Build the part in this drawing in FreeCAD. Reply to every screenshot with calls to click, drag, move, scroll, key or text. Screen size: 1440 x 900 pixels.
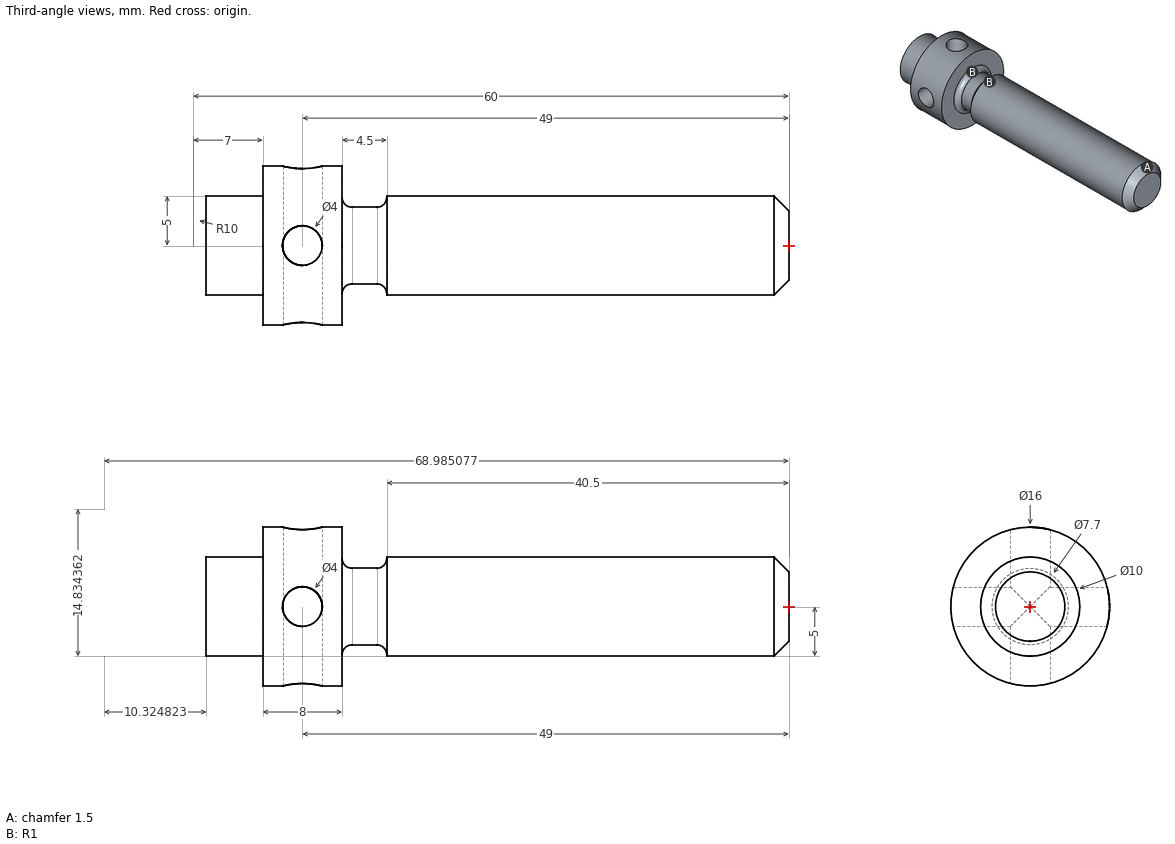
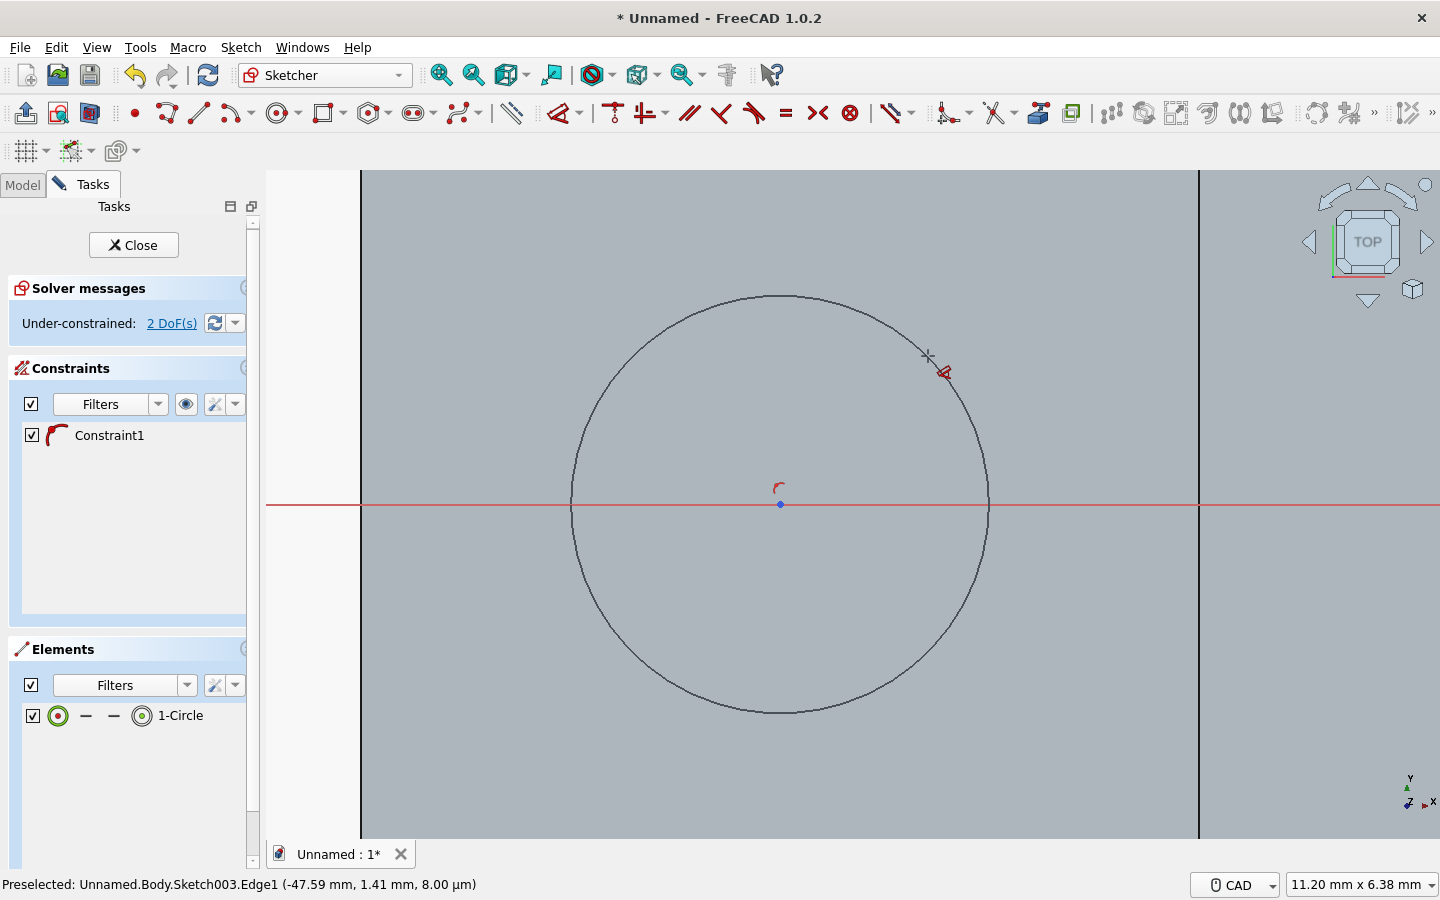
click(927, 356)
click(950, 333)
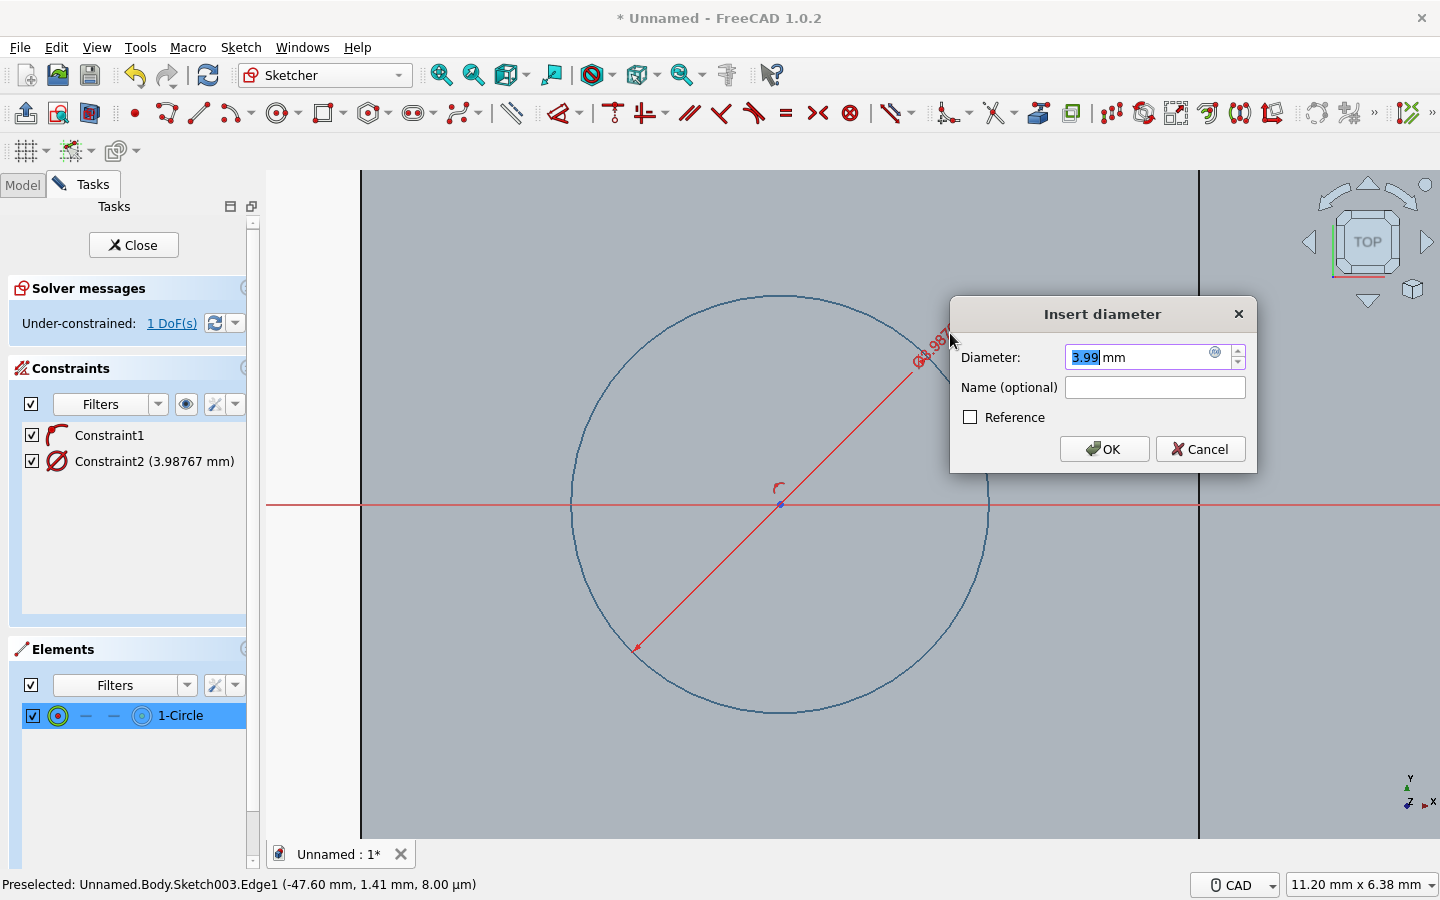
text(4)
key(Return)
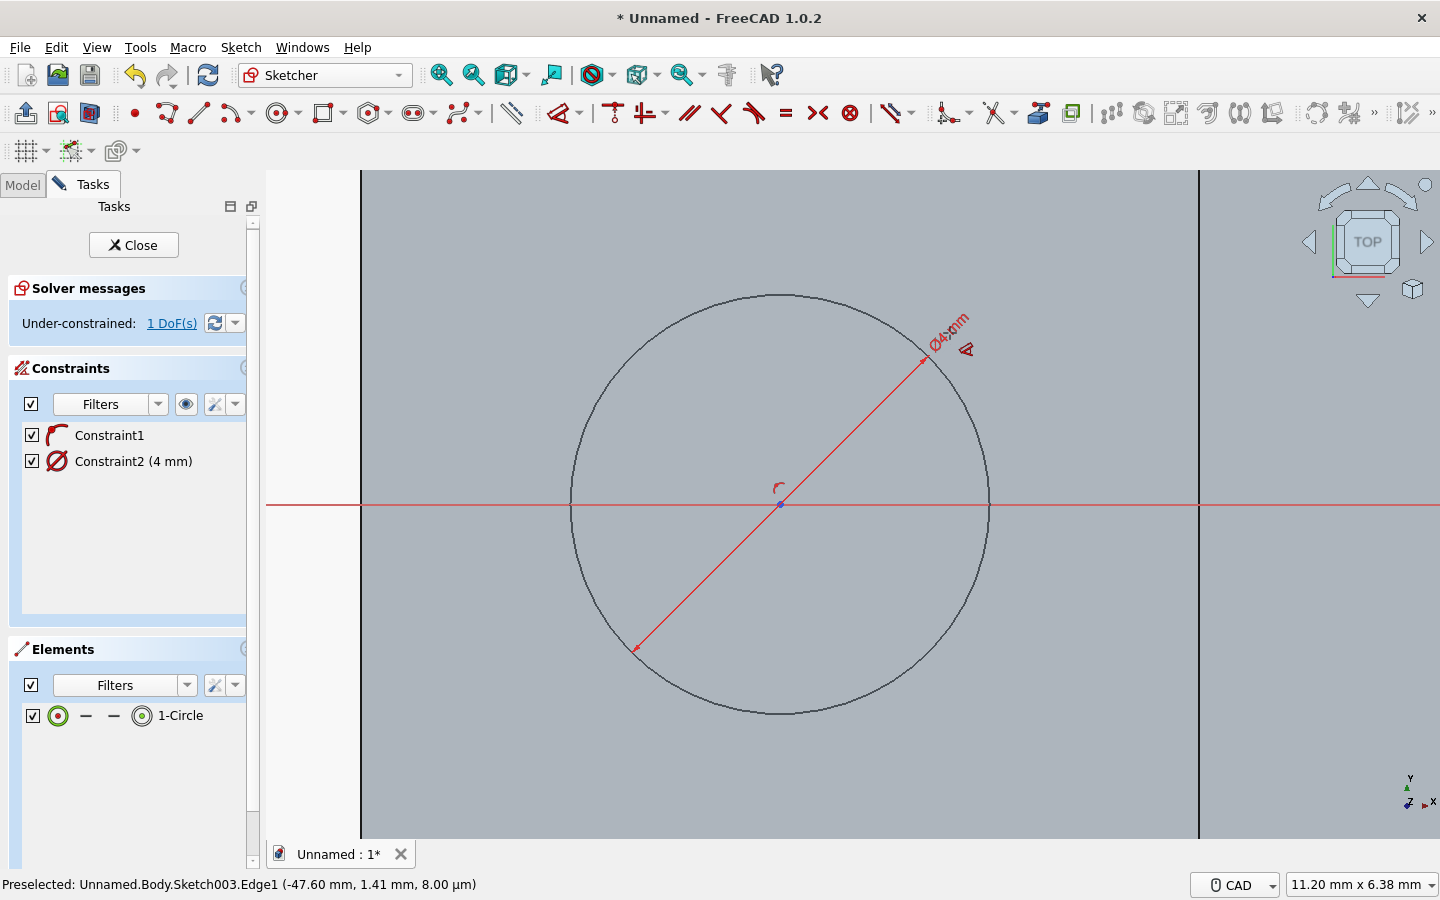
click(780, 504)
click(1027, 538)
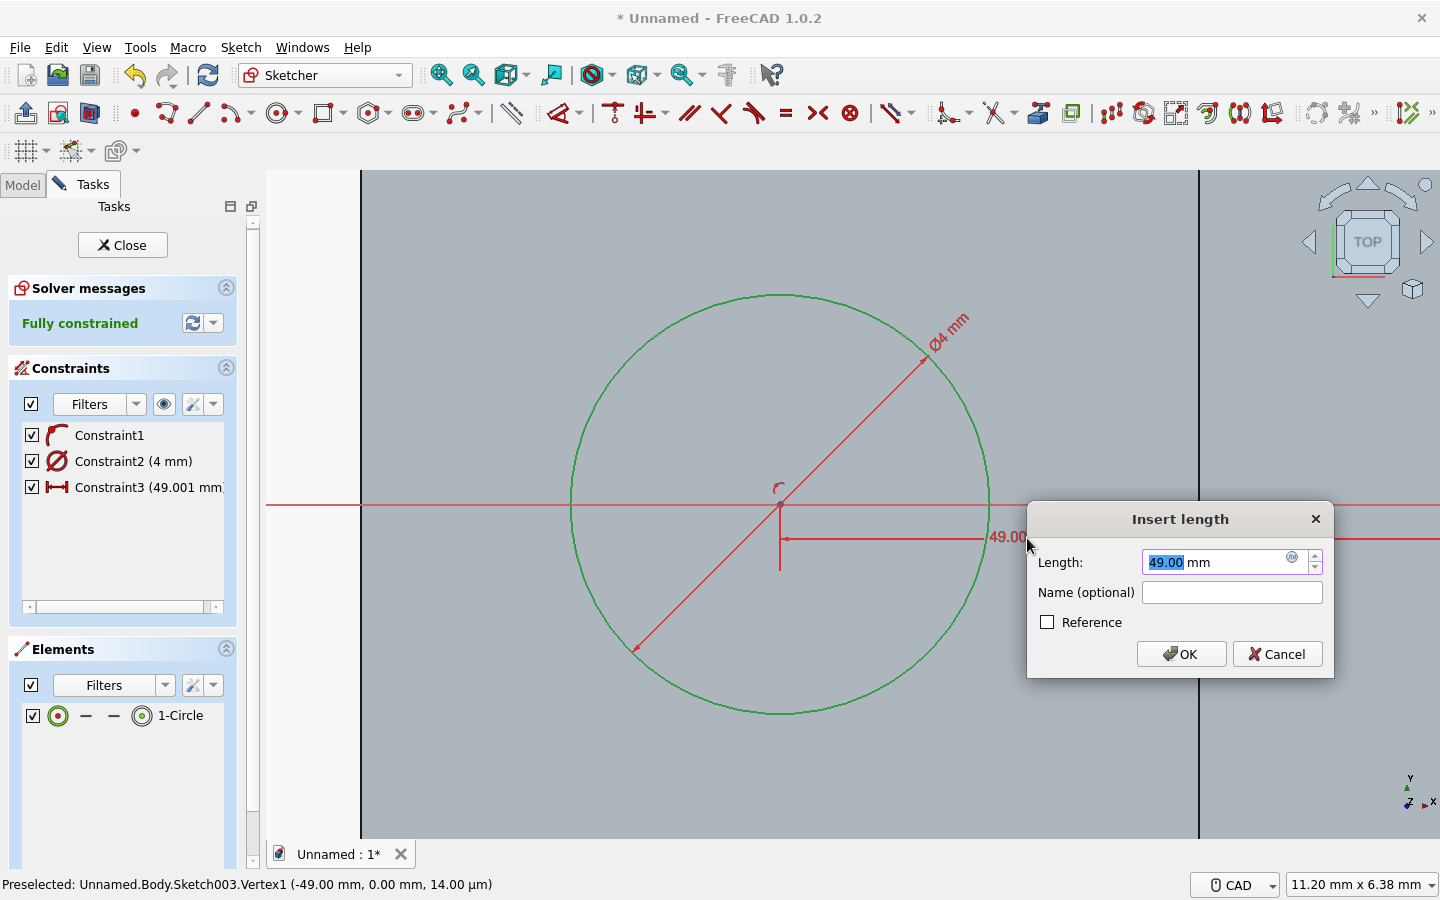
text(49)
key(Return)
key(Escape)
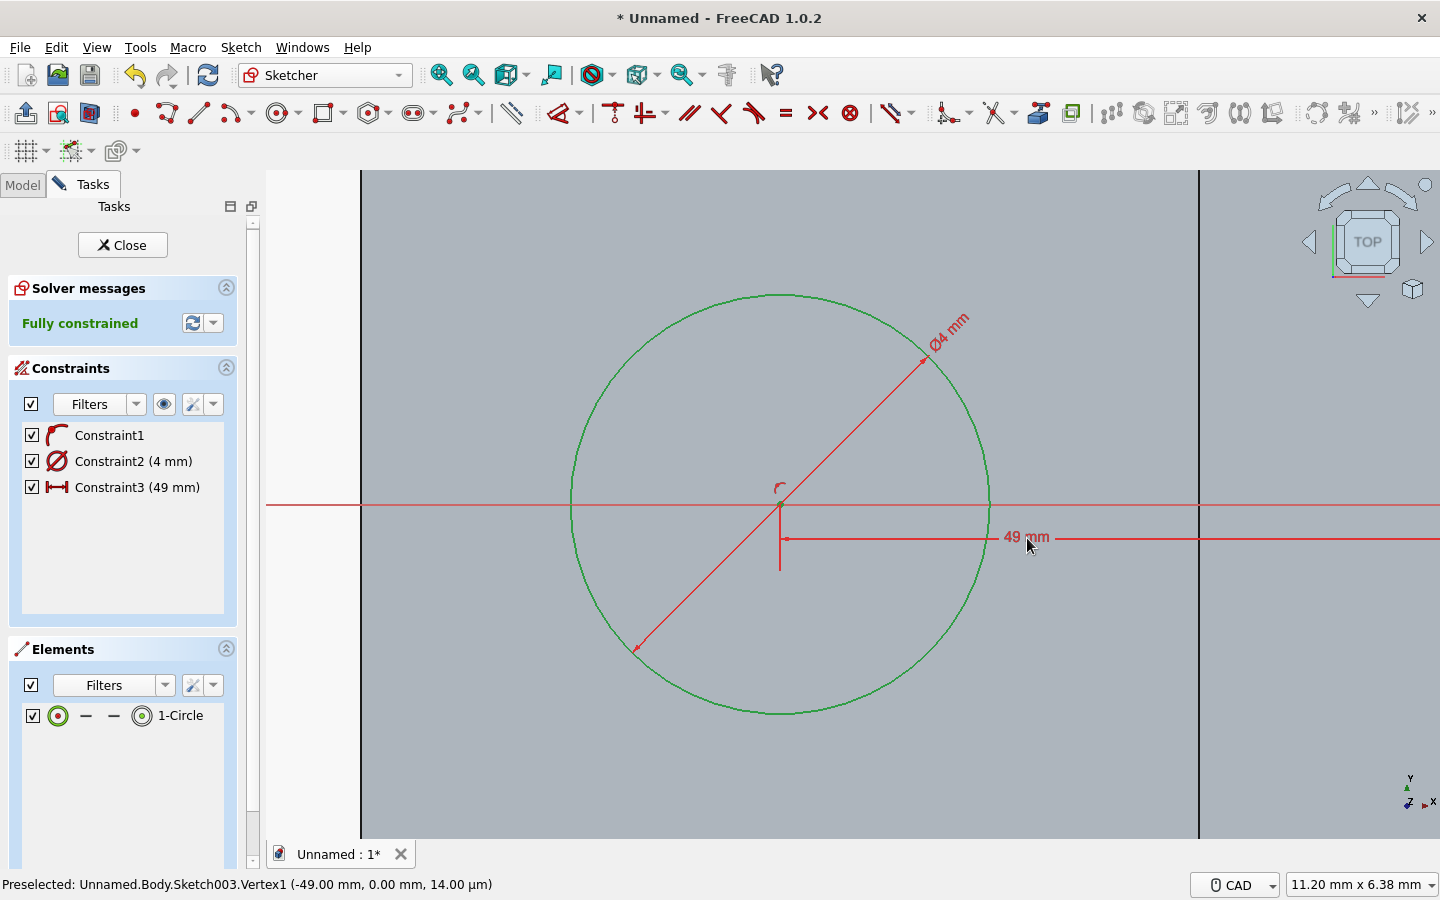
click(123, 245)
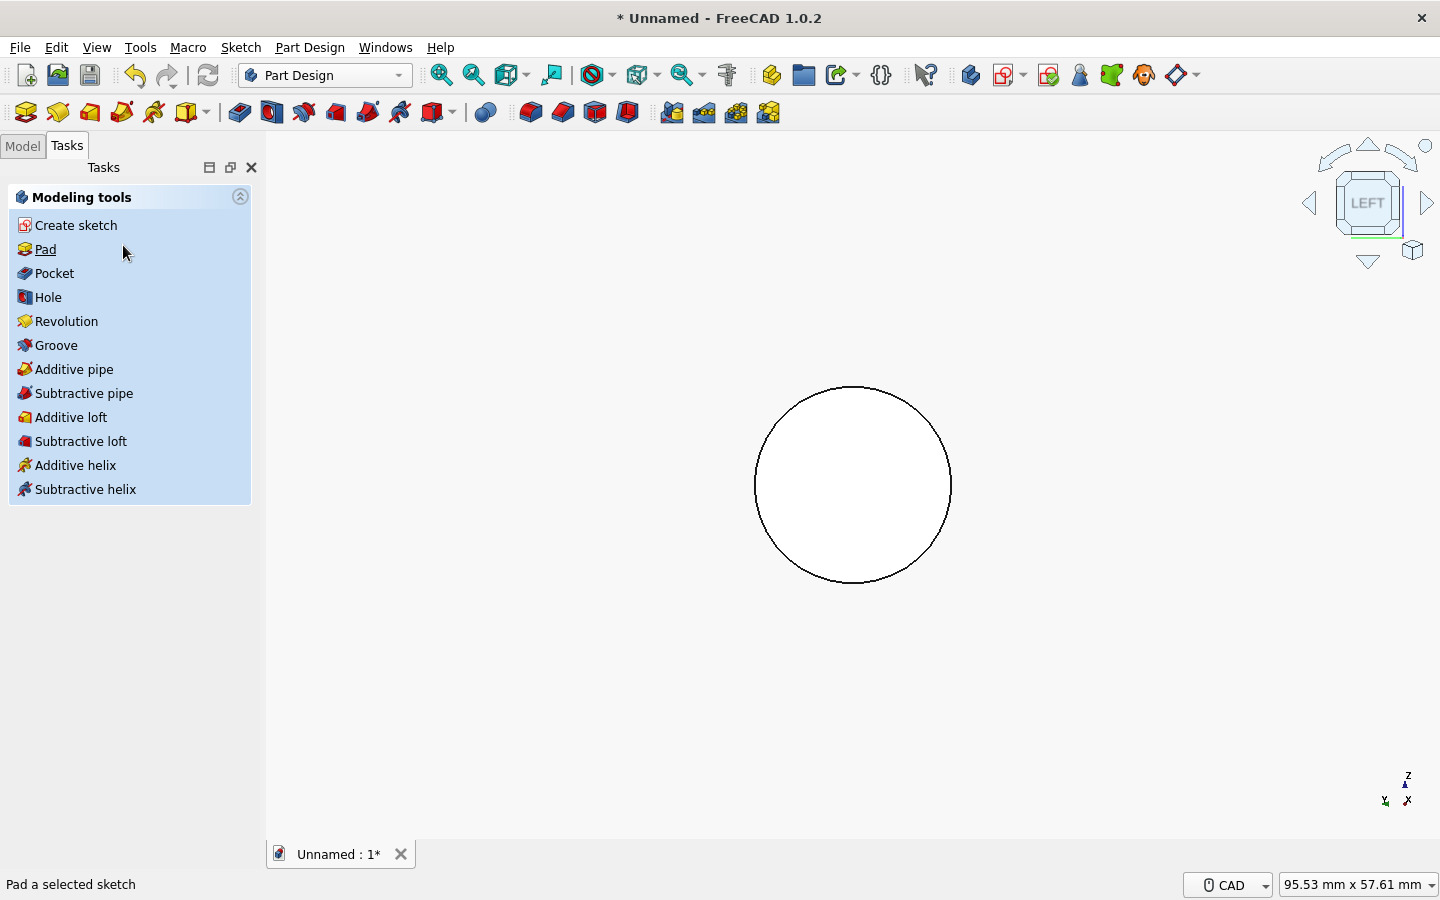
click(240, 112)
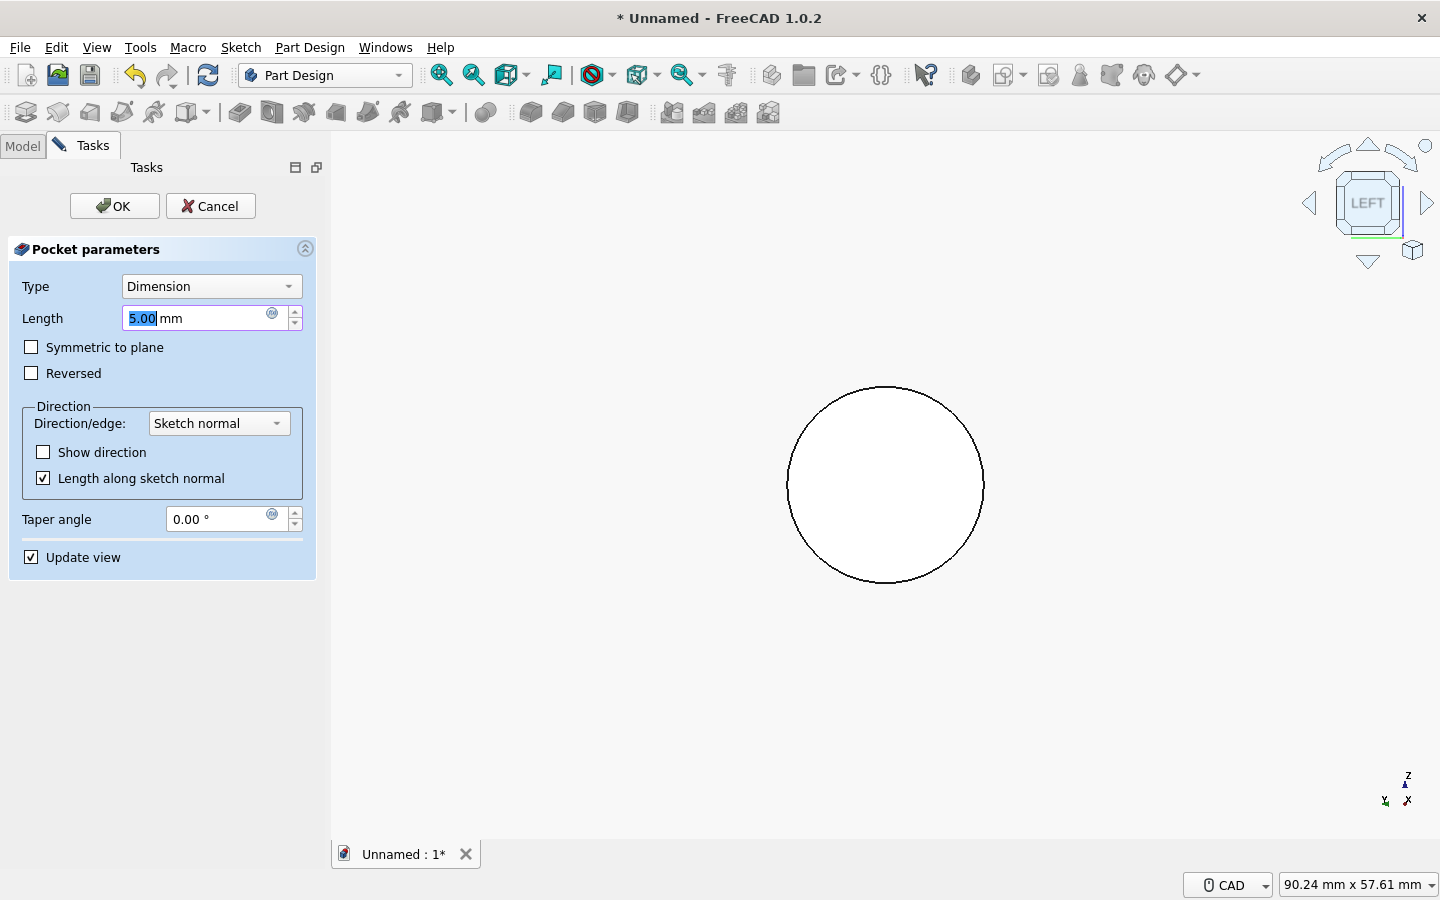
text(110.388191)
key(Tab)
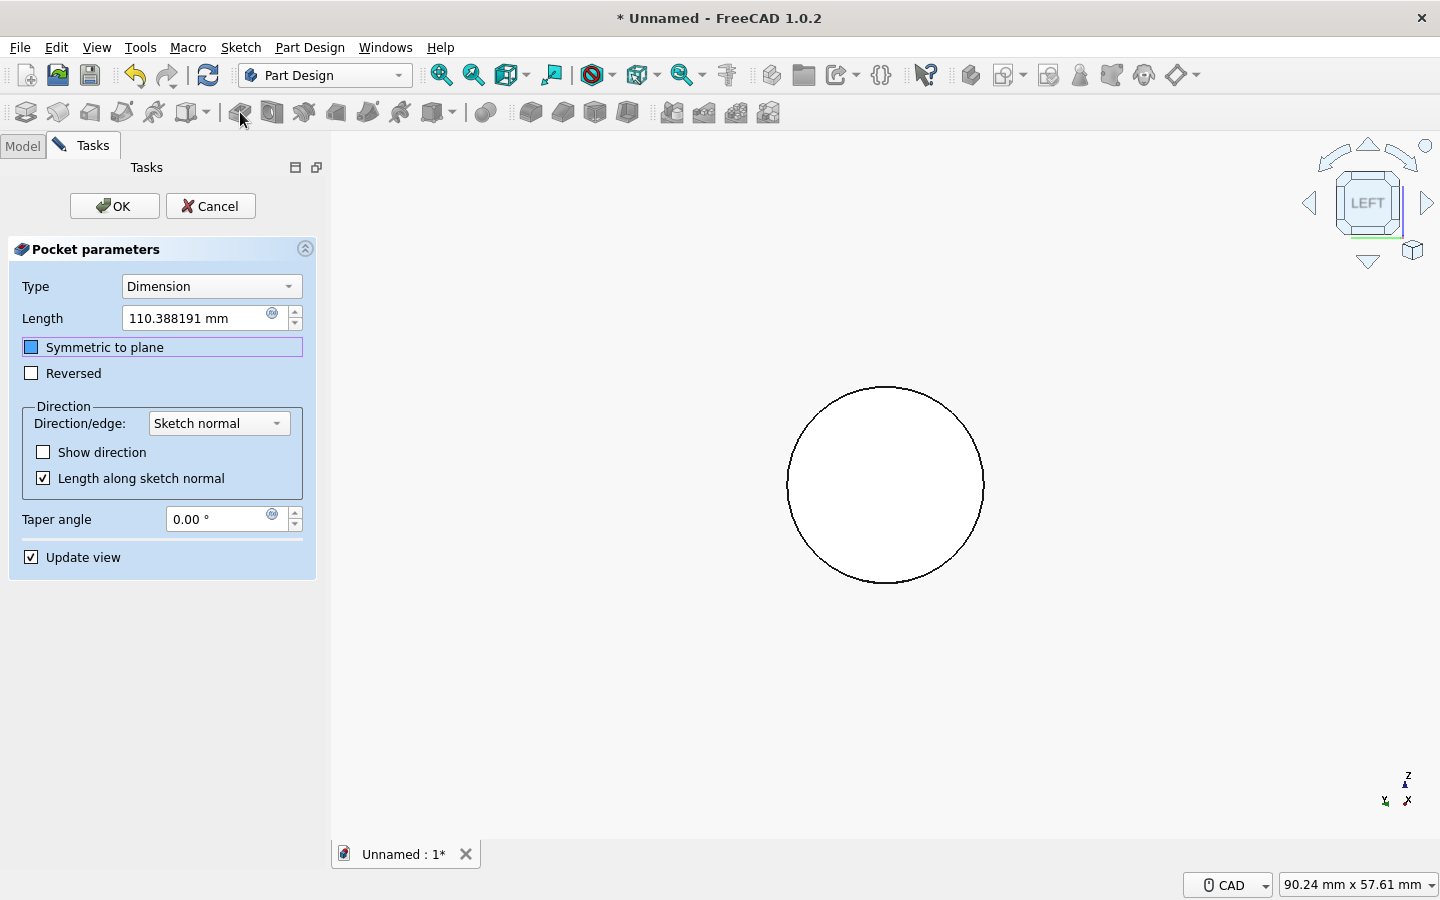
click(30, 347)